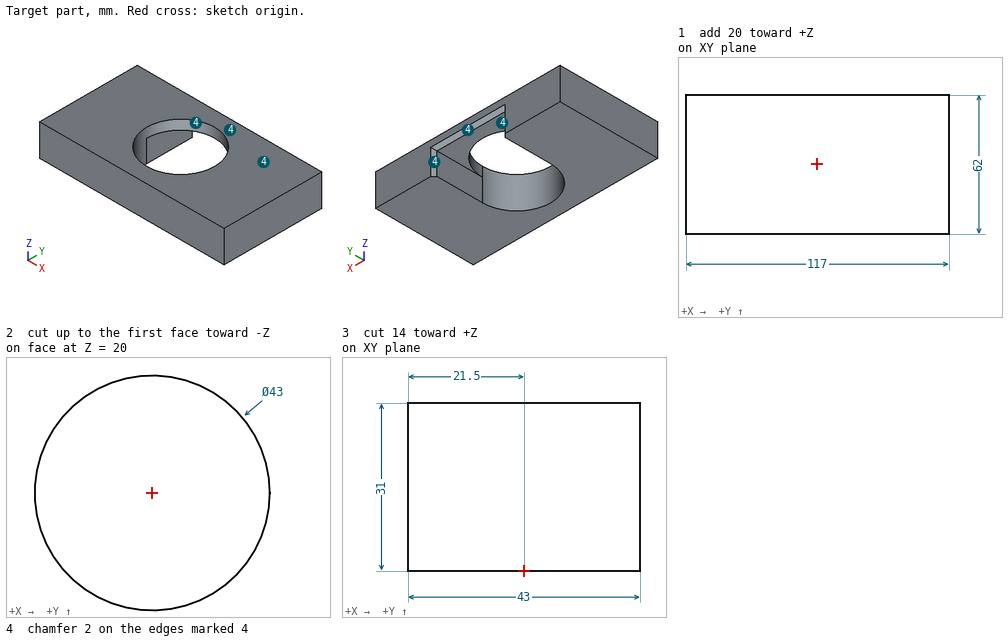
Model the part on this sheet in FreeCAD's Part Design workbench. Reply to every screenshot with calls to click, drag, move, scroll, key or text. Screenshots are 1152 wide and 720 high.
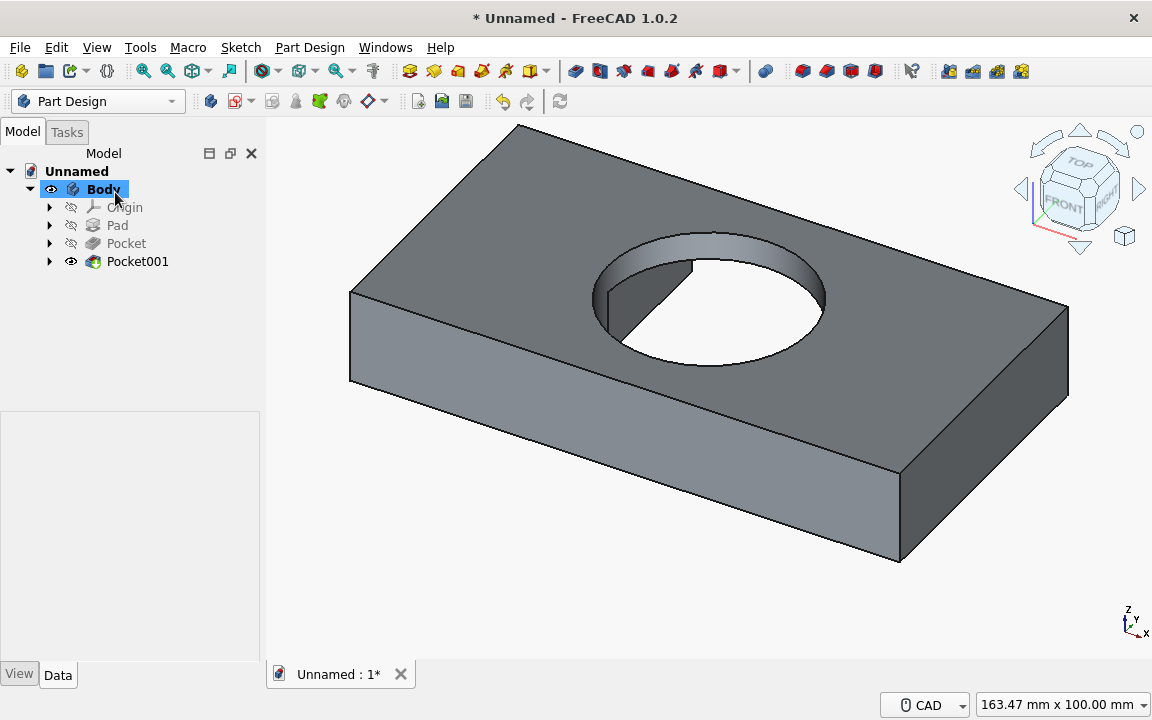
key(0)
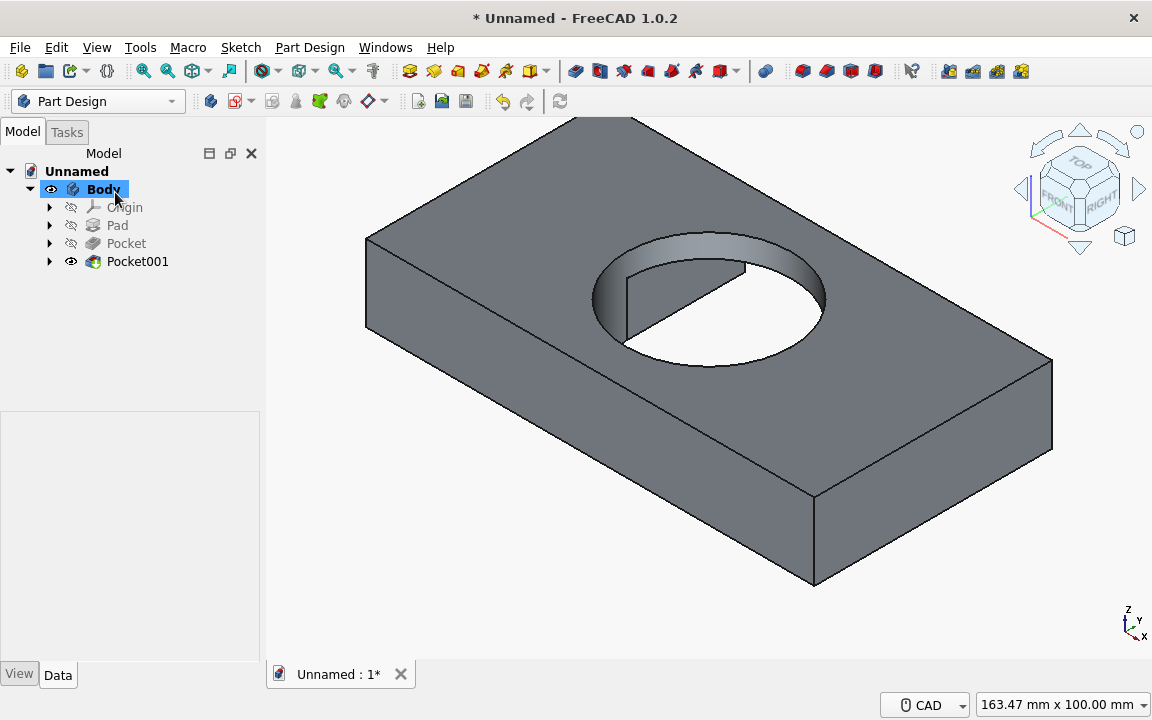
key(v)
key(f)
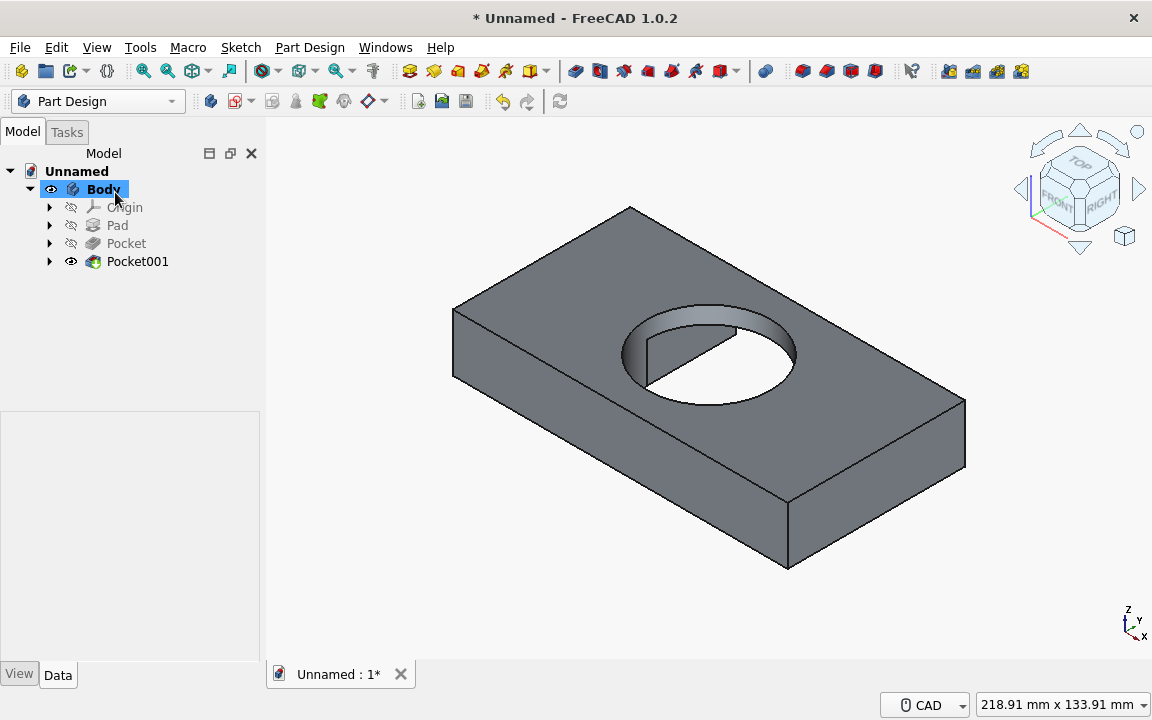
key(2)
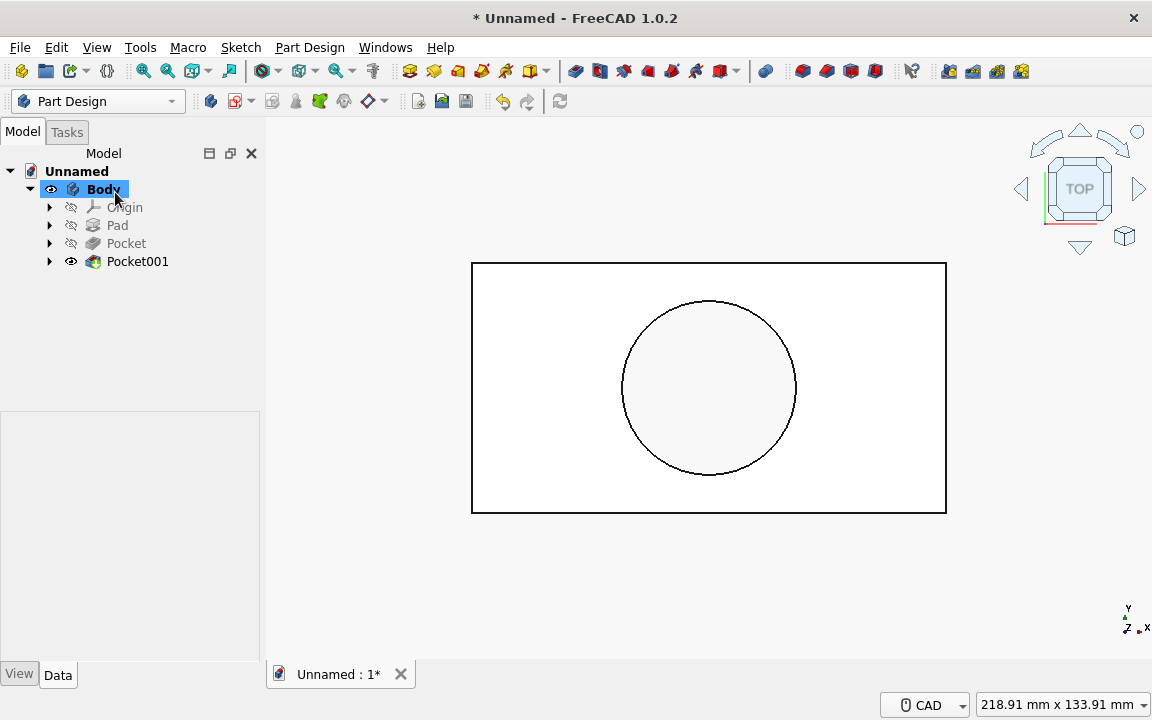
key(1)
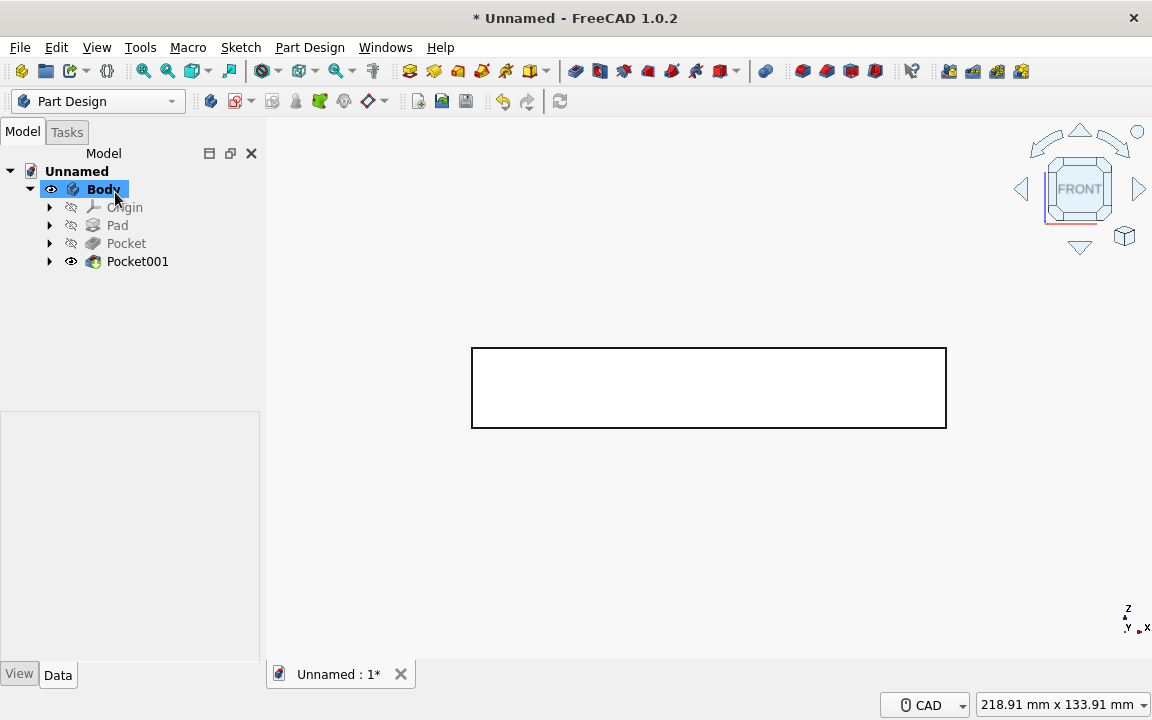
key(3)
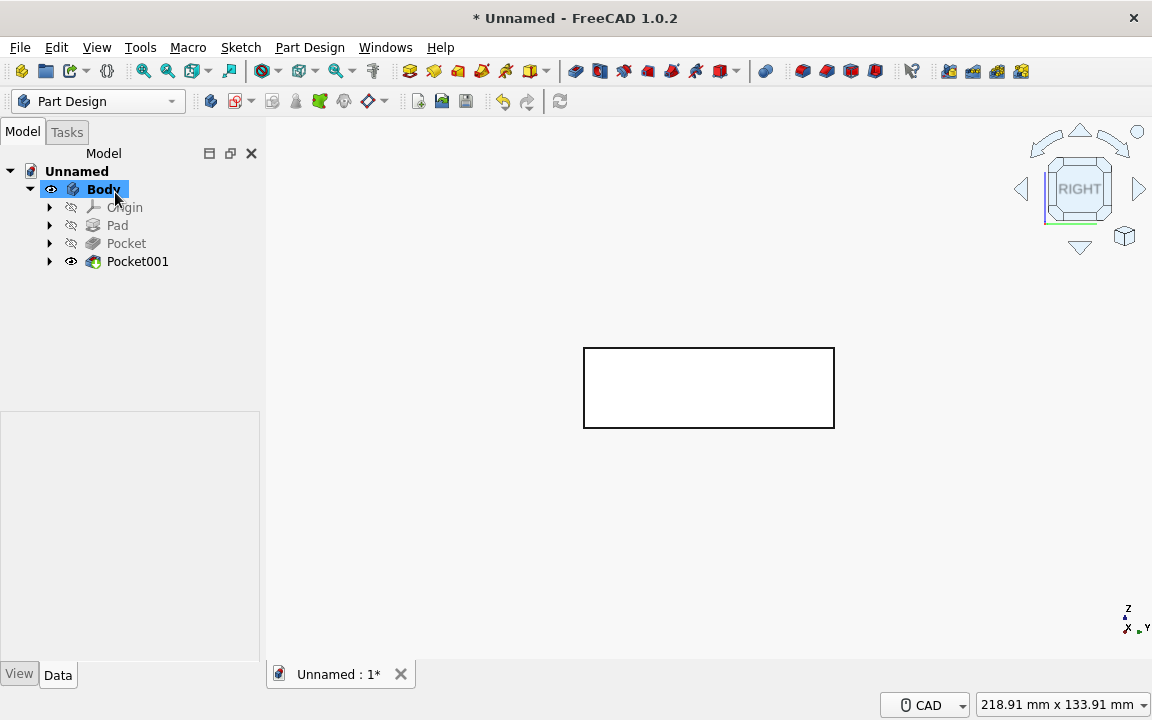
click(144, 72)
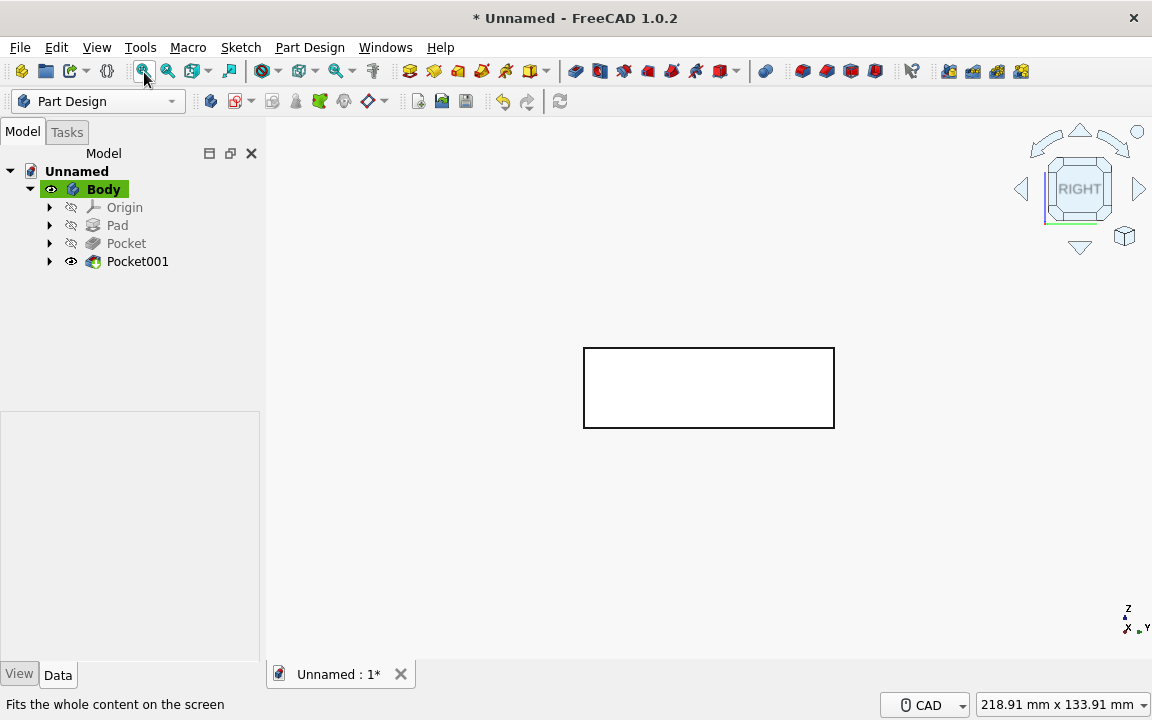
key(5)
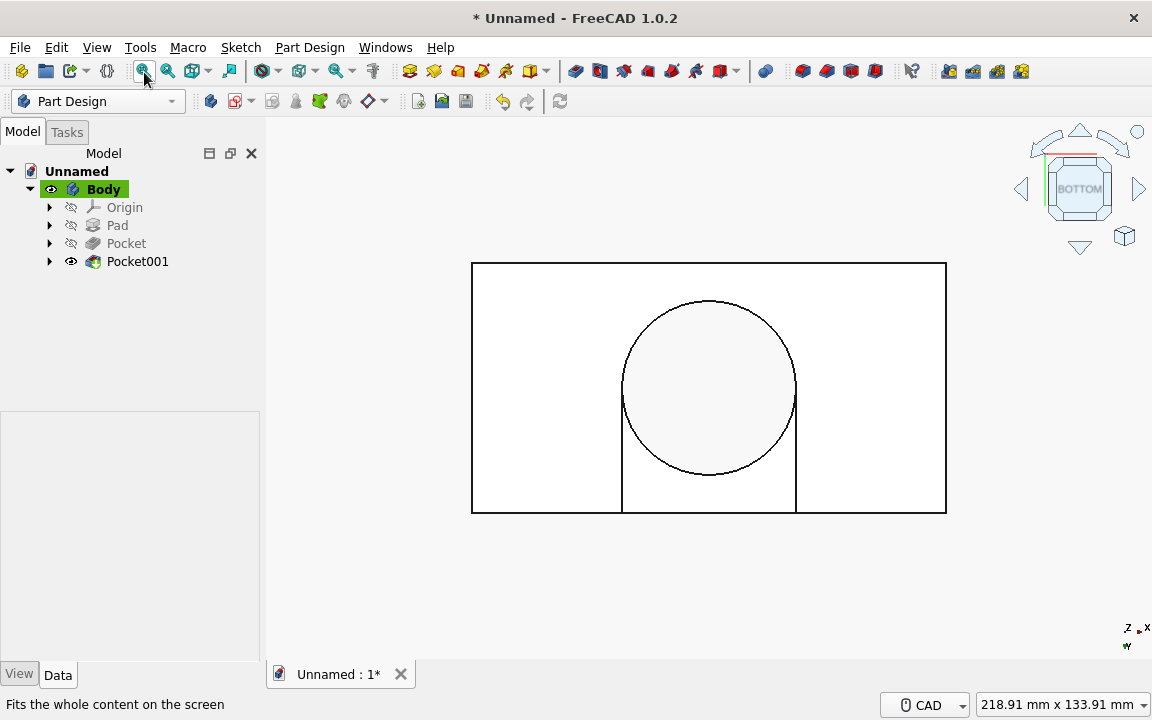
click(709, 512)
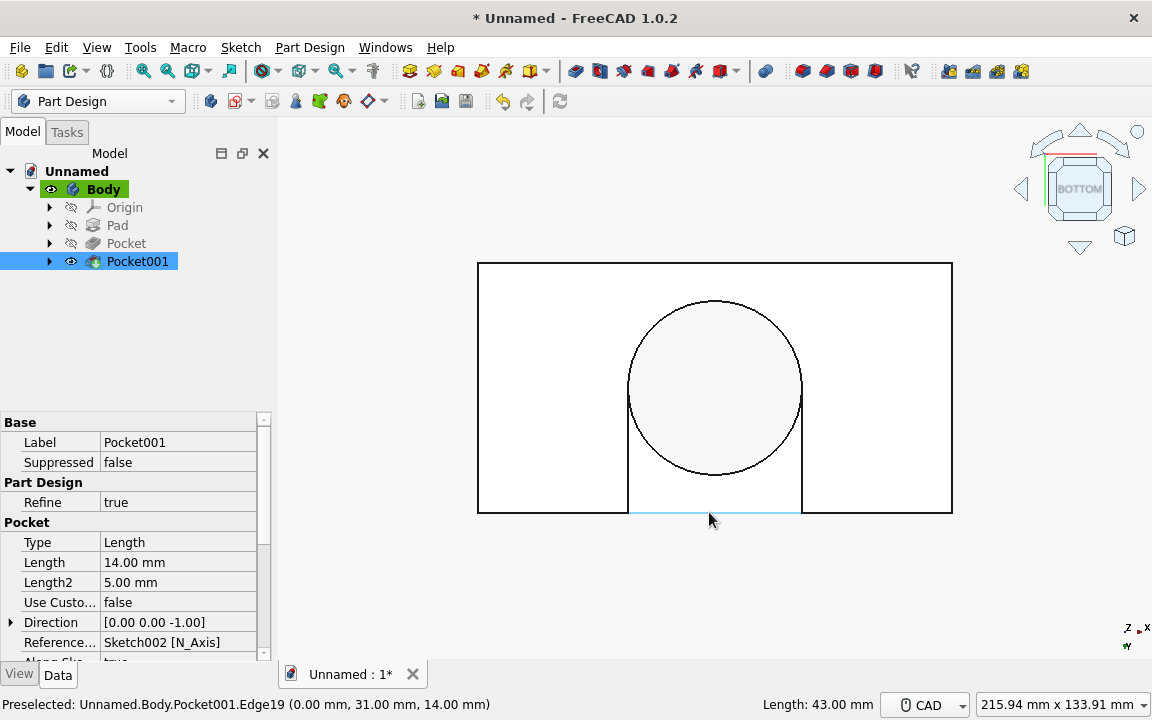
key(4)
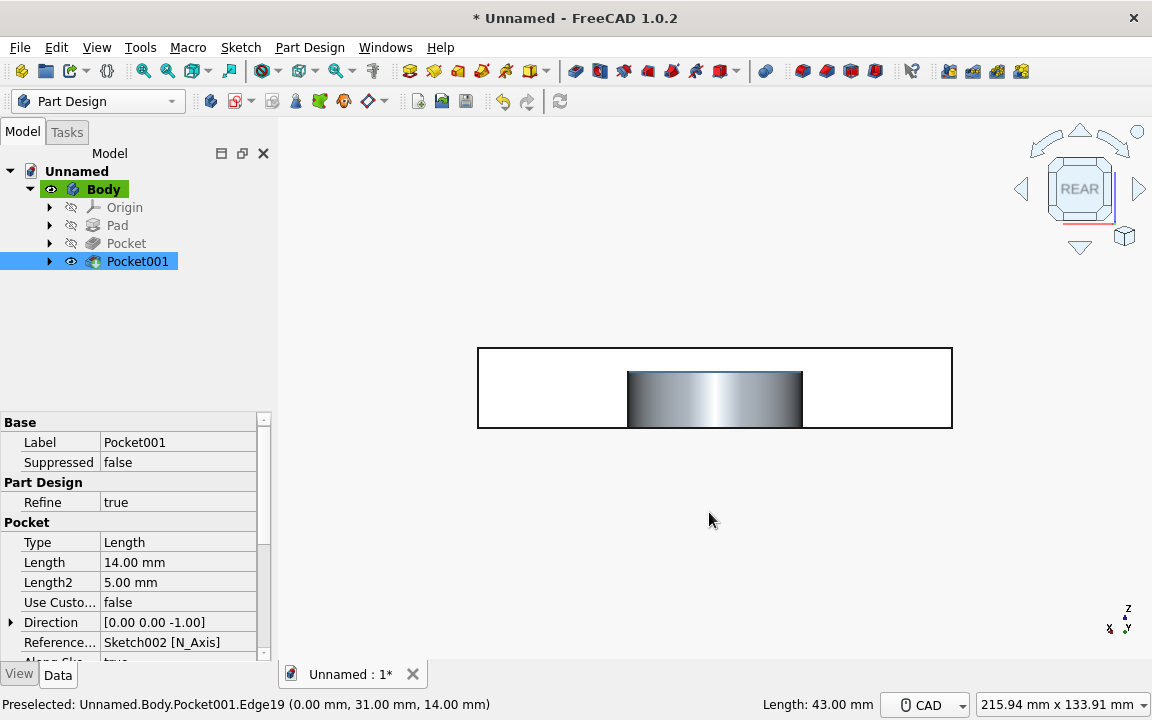
click(628, 399, ctrl)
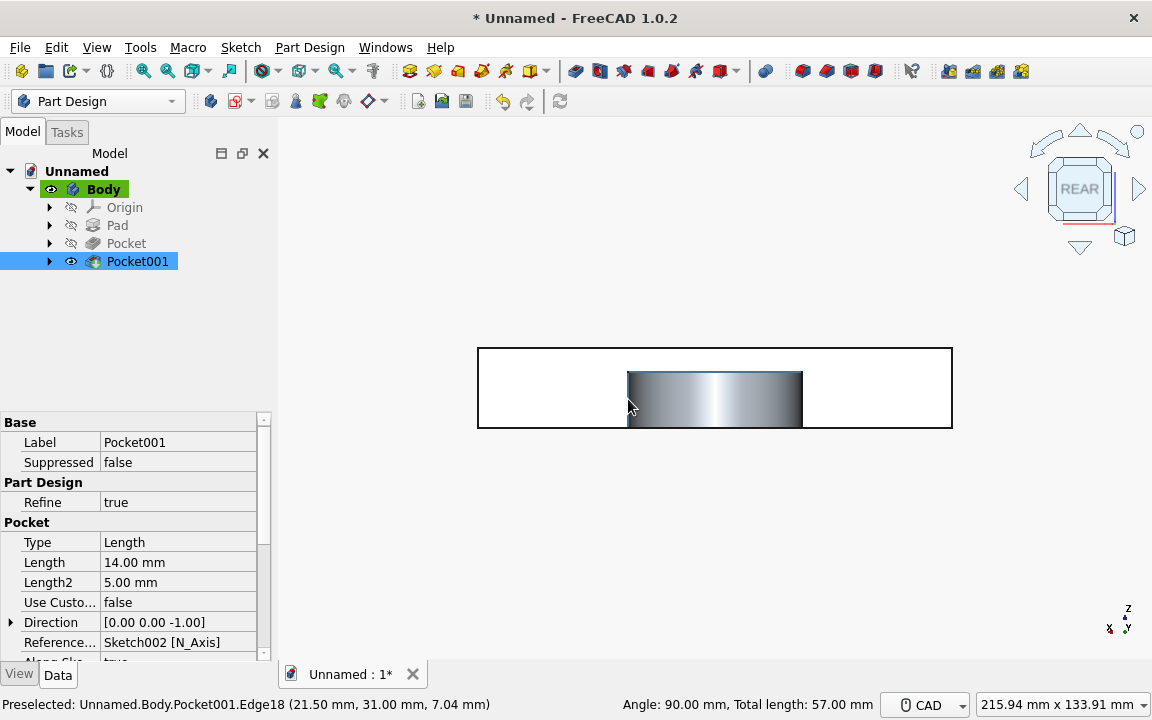
click(802, 399, ctrl)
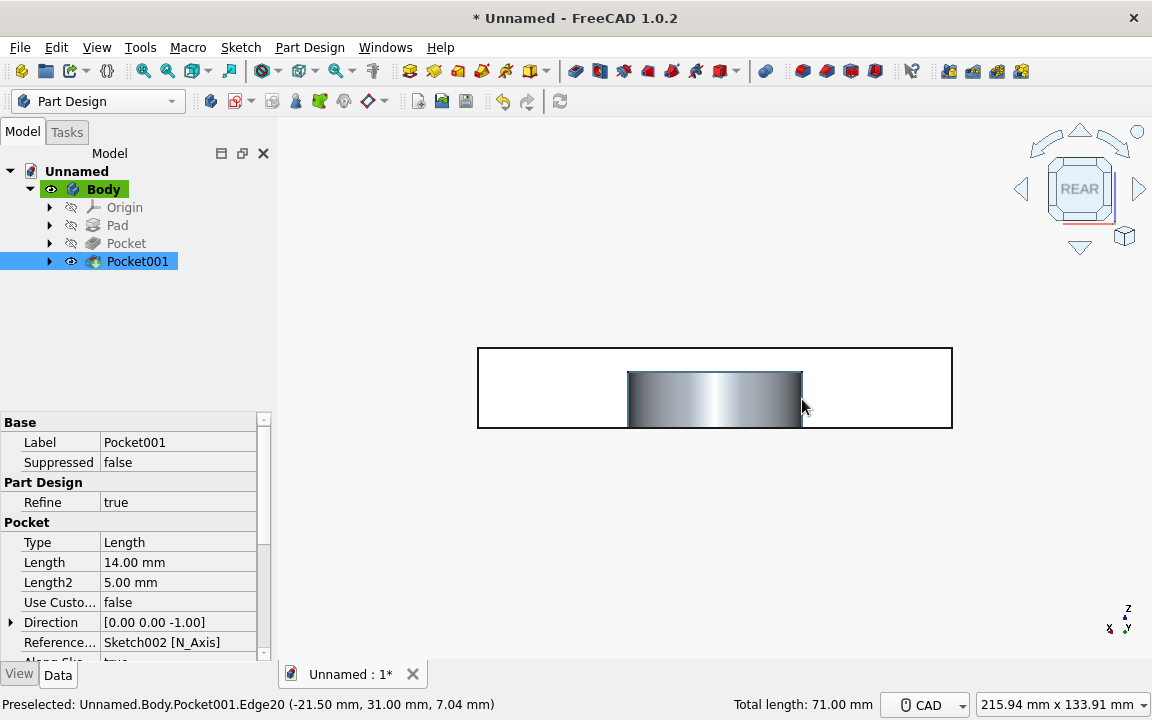
click(828, 72)